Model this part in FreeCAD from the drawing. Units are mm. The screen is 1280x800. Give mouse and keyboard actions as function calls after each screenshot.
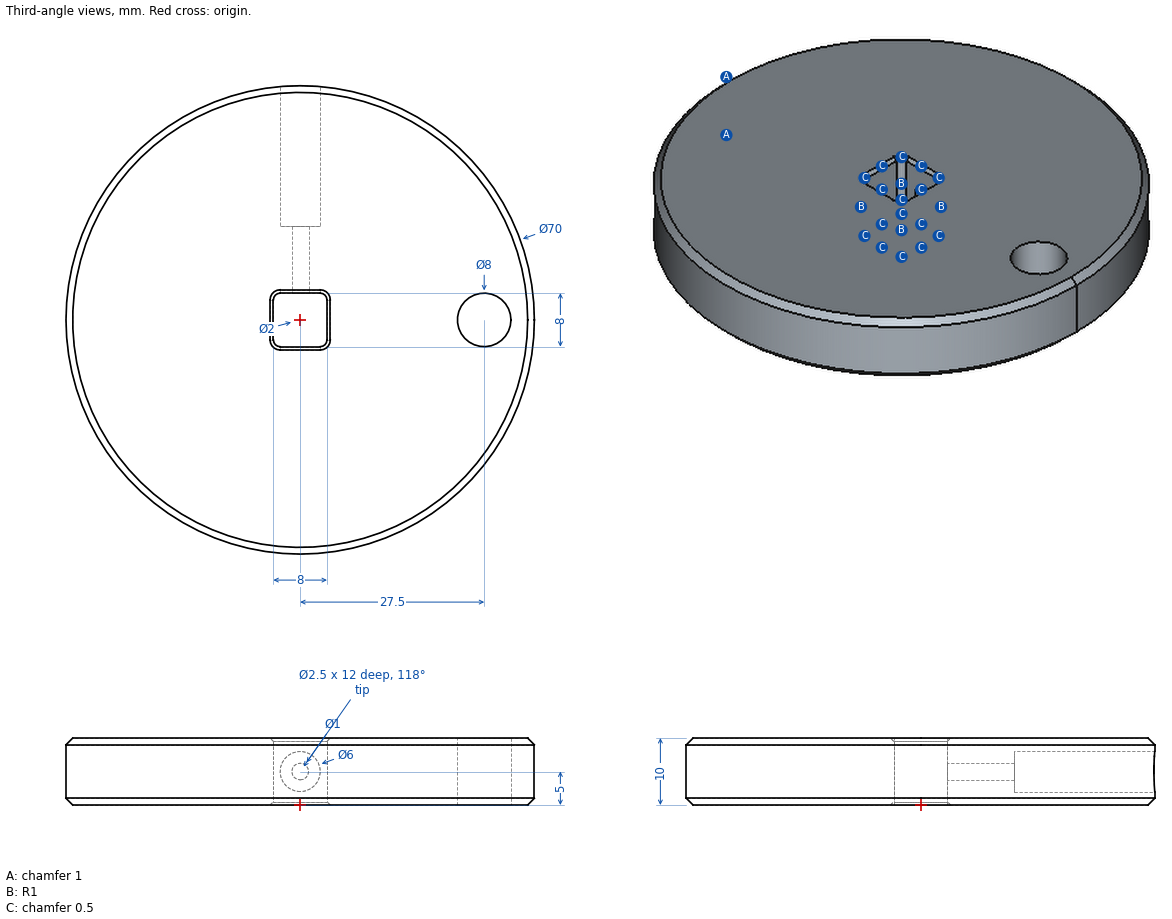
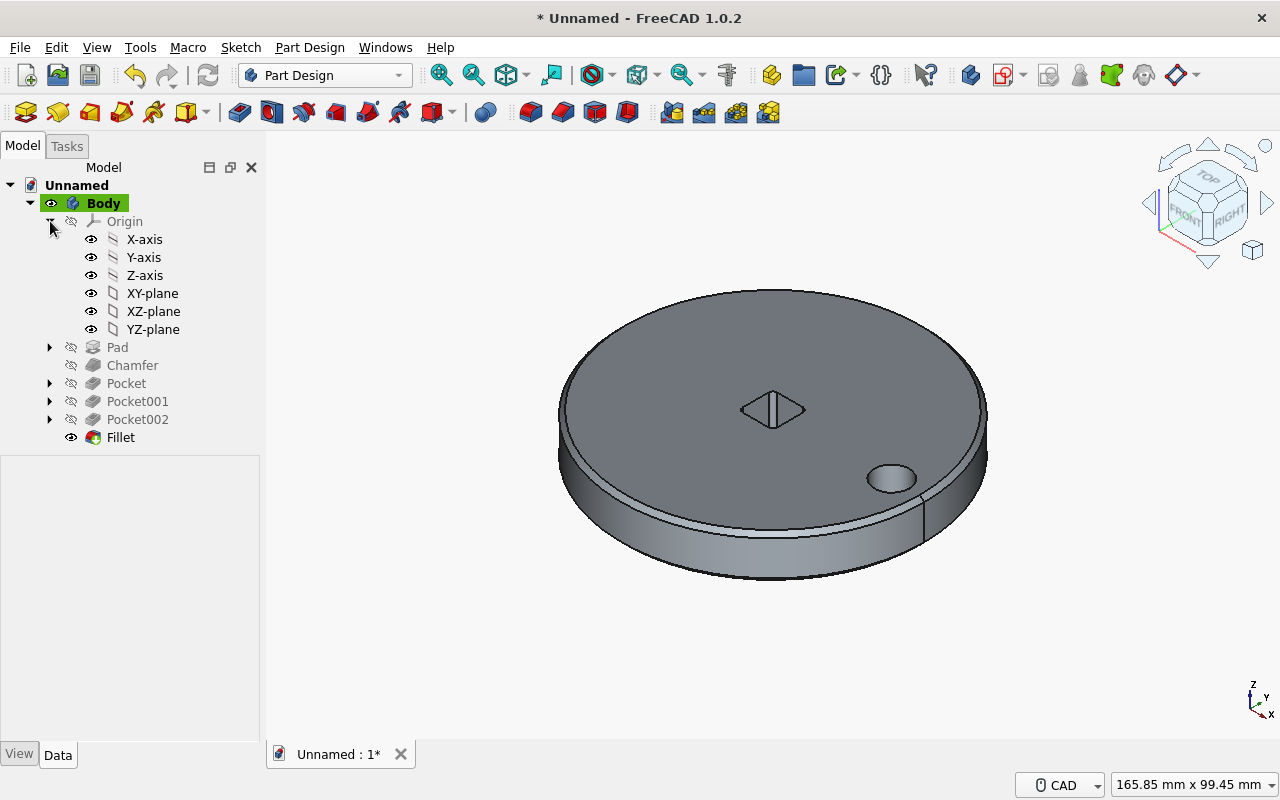
click(136, 311)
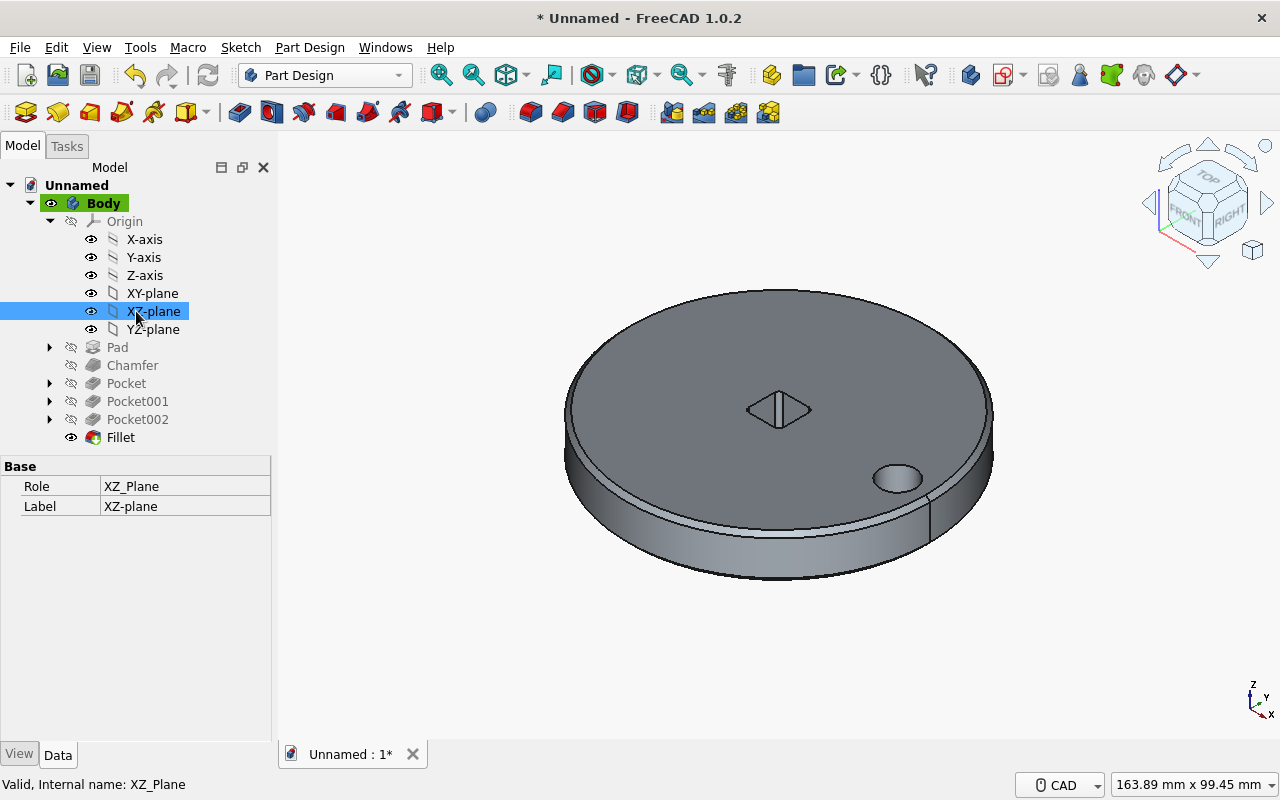
click(1176, 76)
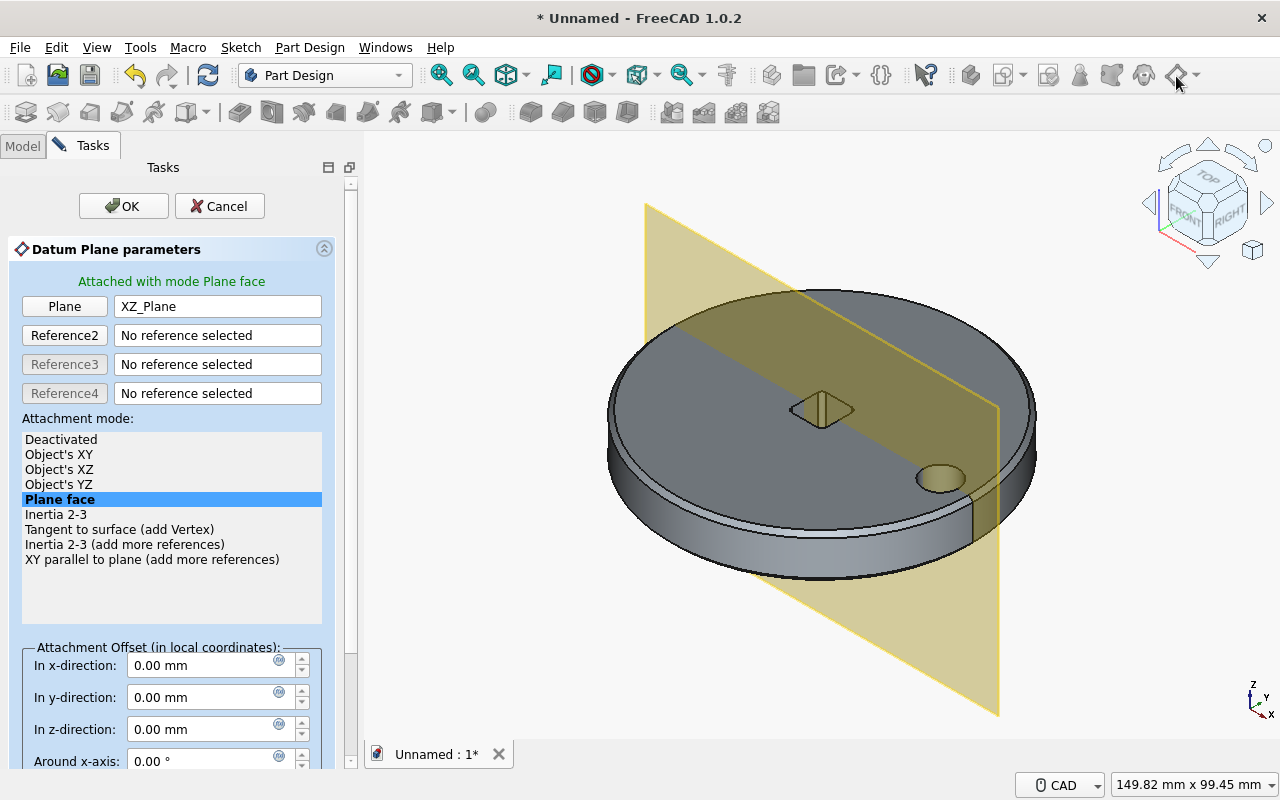
triple_click(210, 729)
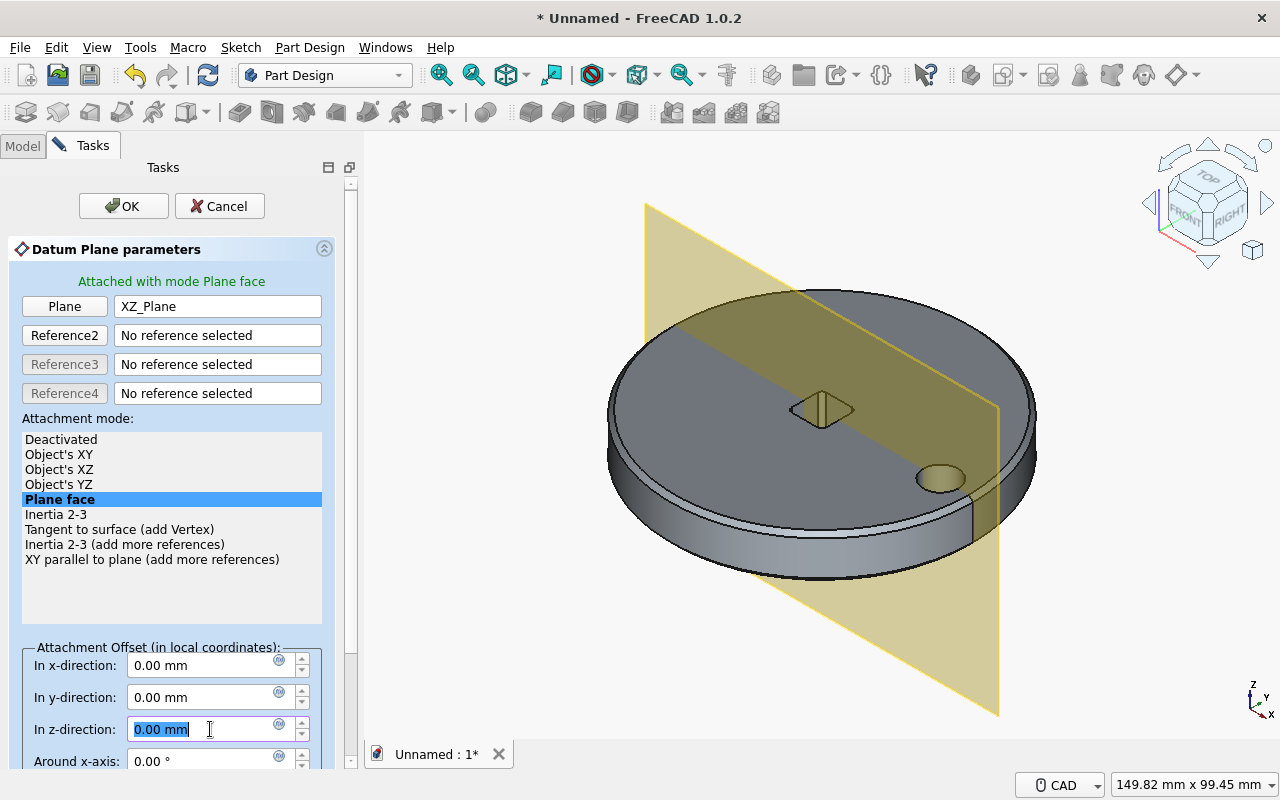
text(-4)
key(Tab)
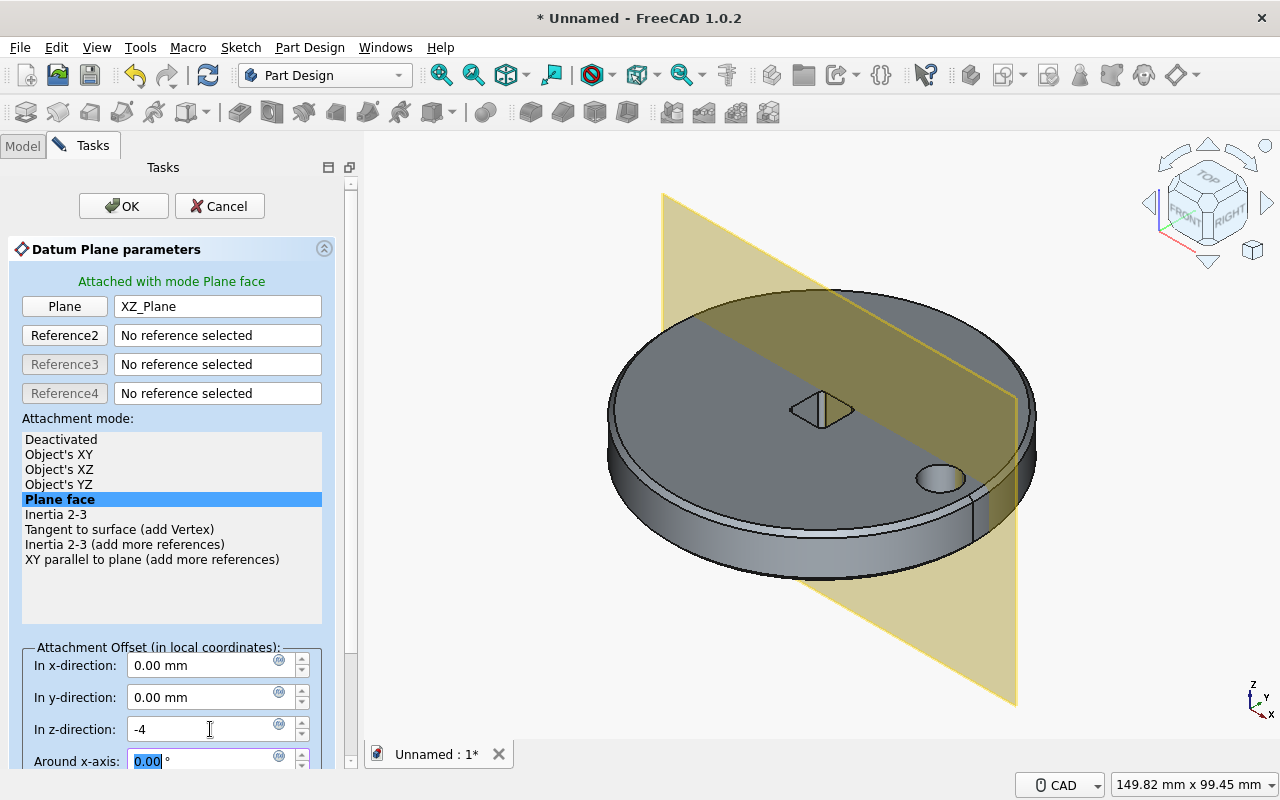
click(124, 206)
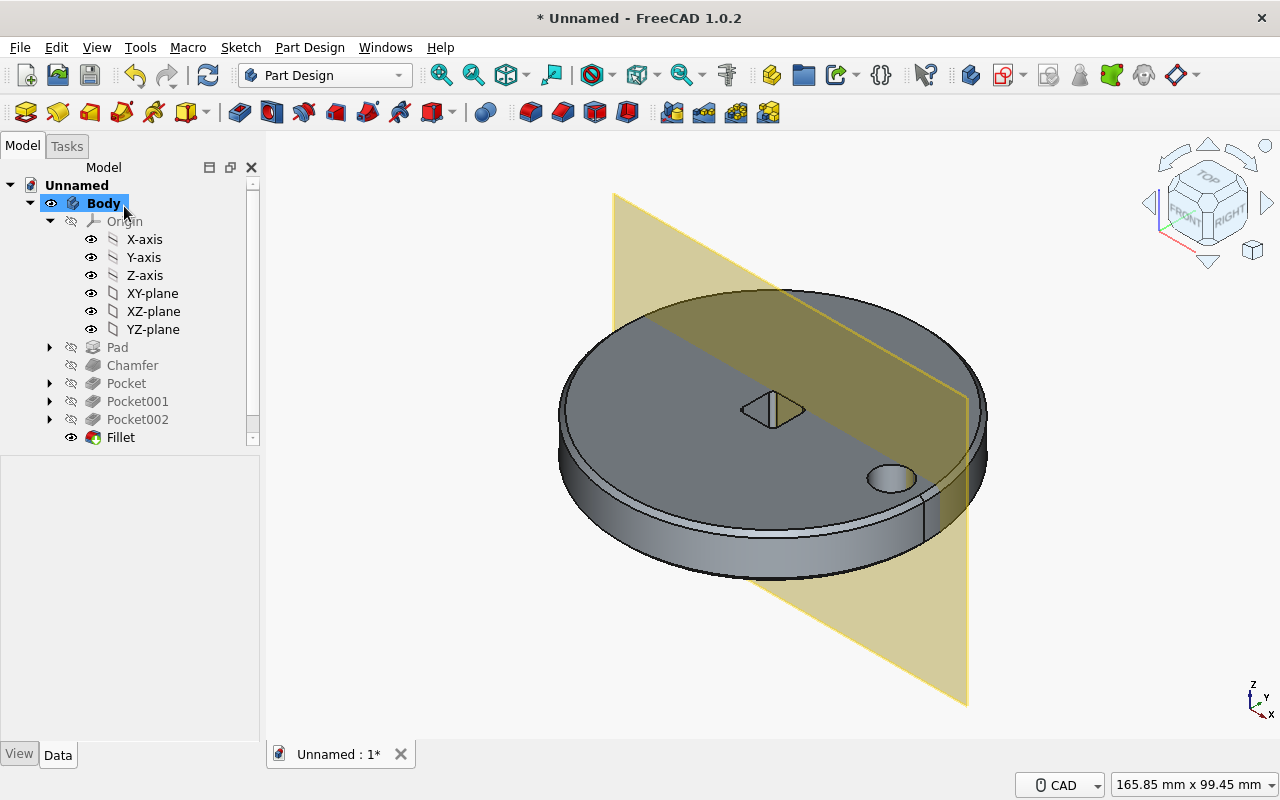
scroll(100, 307, down, 3)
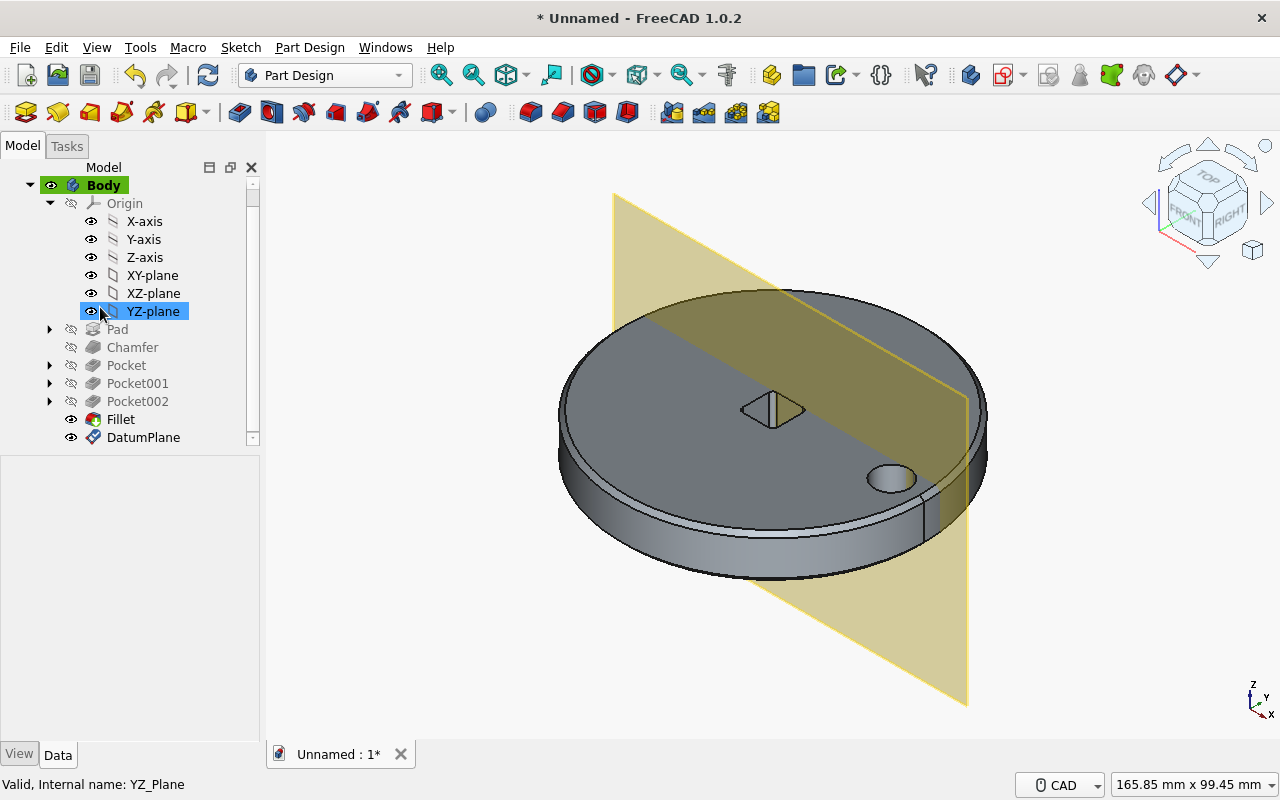
click(116, 437)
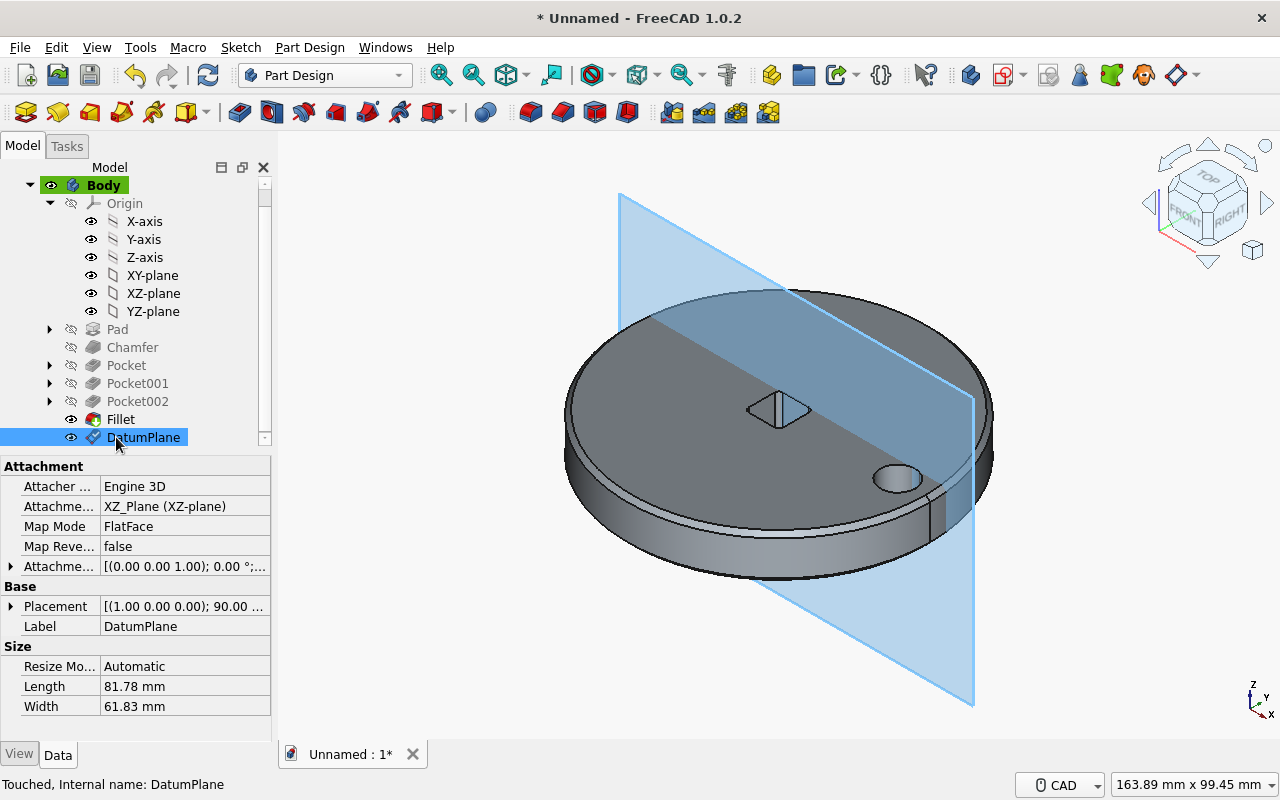
click(1004, 76)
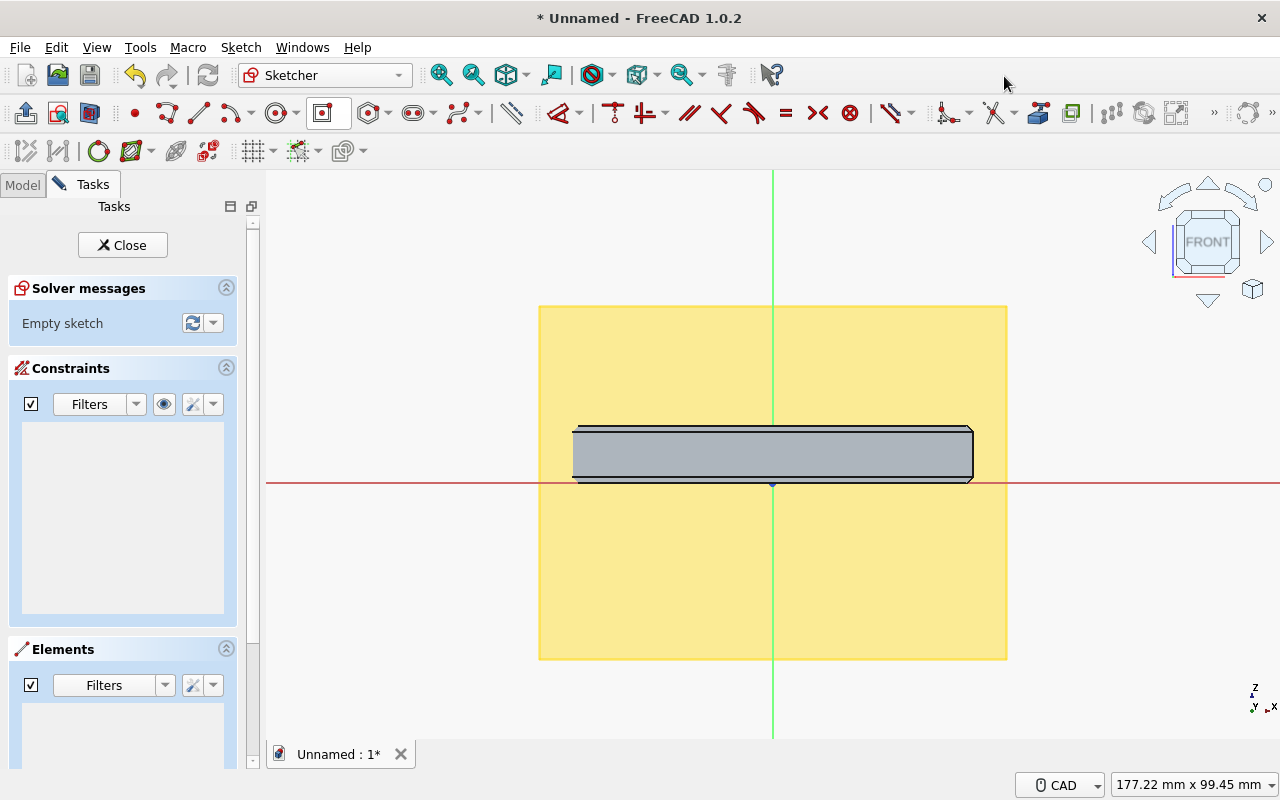
key(q)
key(s)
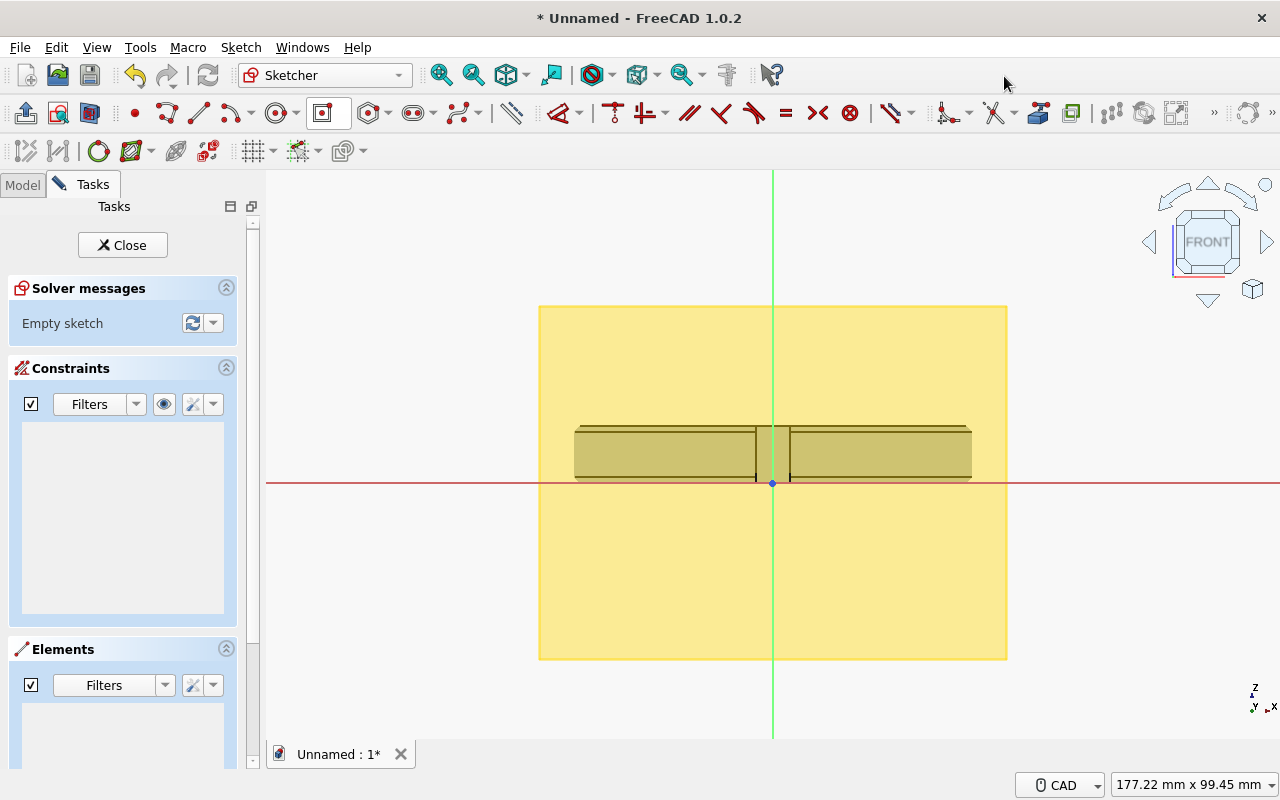
scroll(776, 455, up, 15)